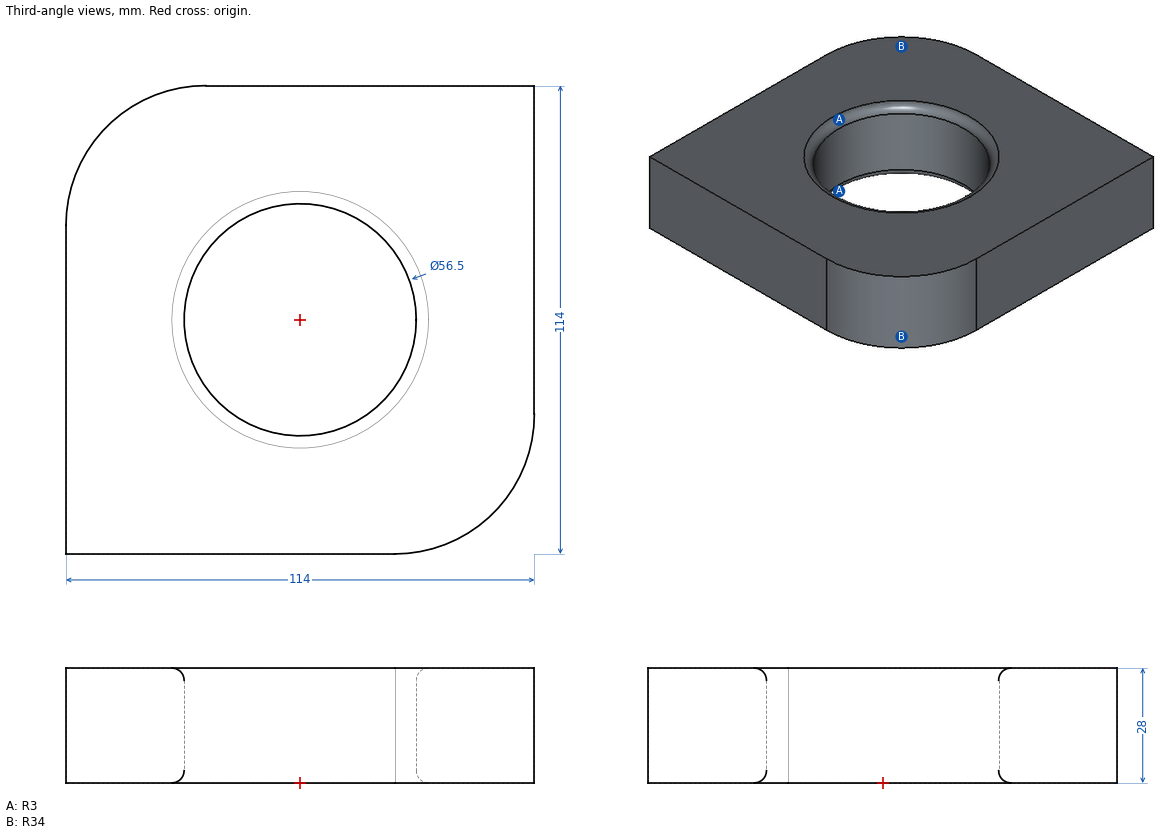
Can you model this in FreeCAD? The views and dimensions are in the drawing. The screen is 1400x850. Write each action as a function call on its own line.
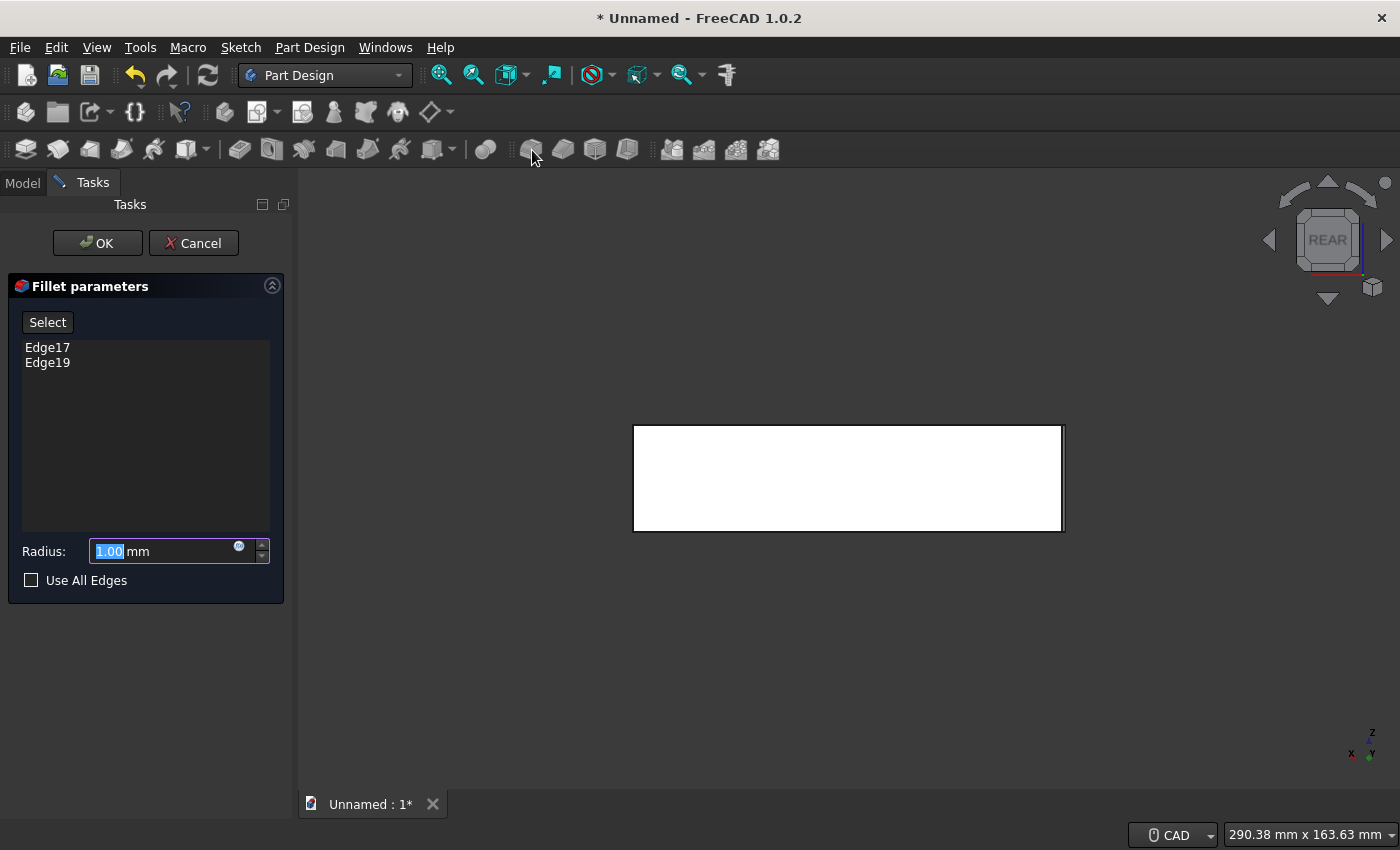
text(34)
key(Tab)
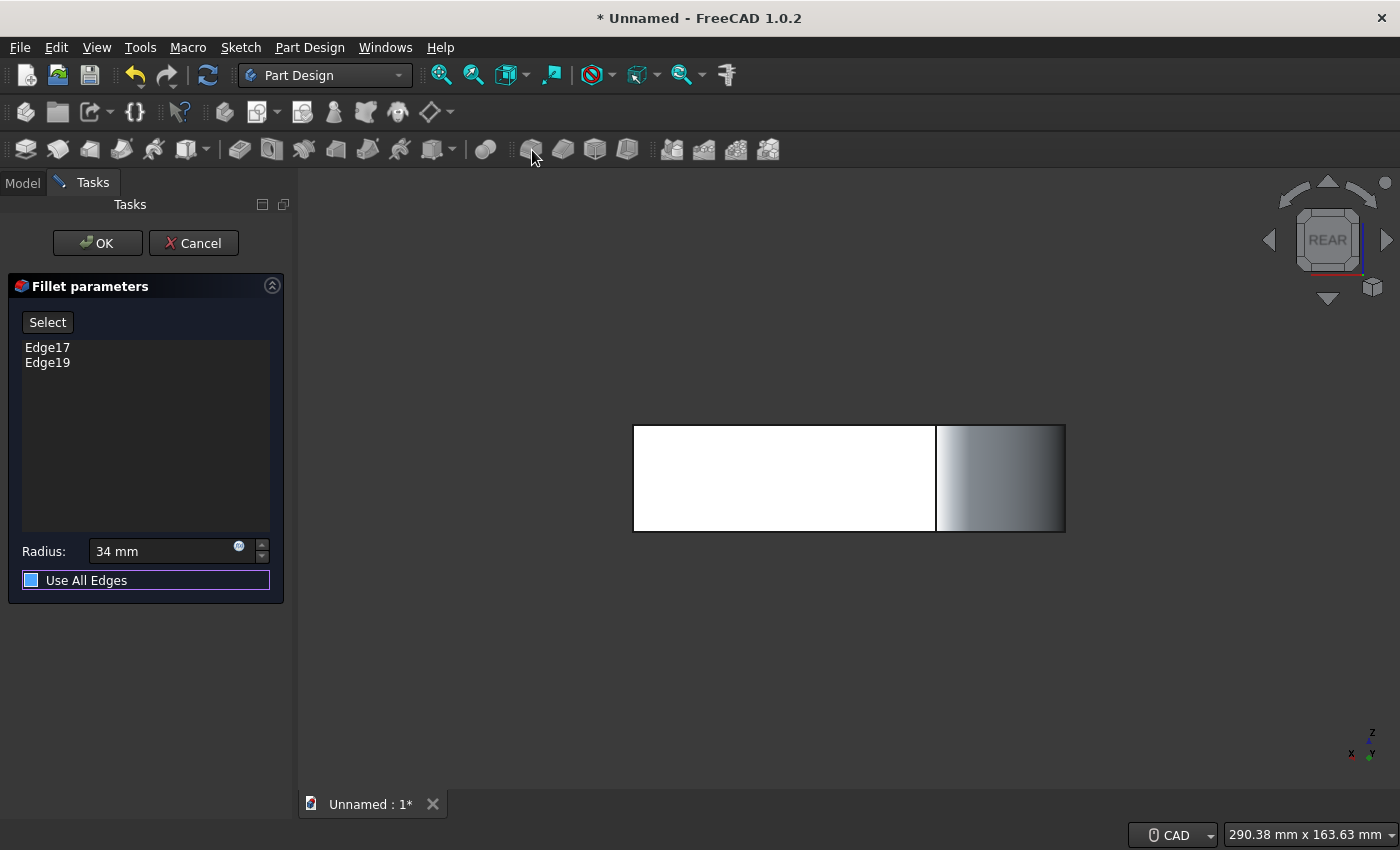
click(98, 243)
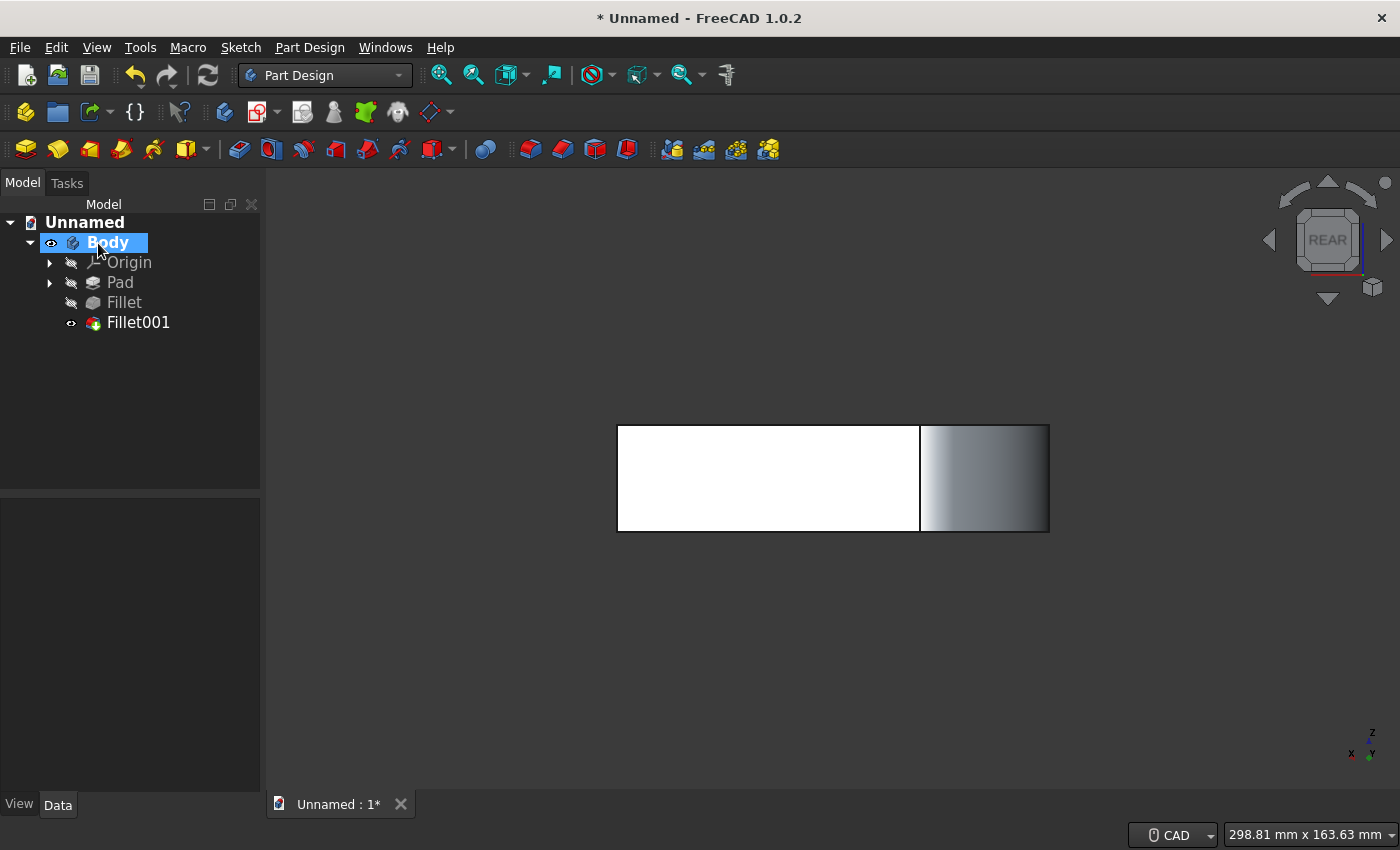
key(0)